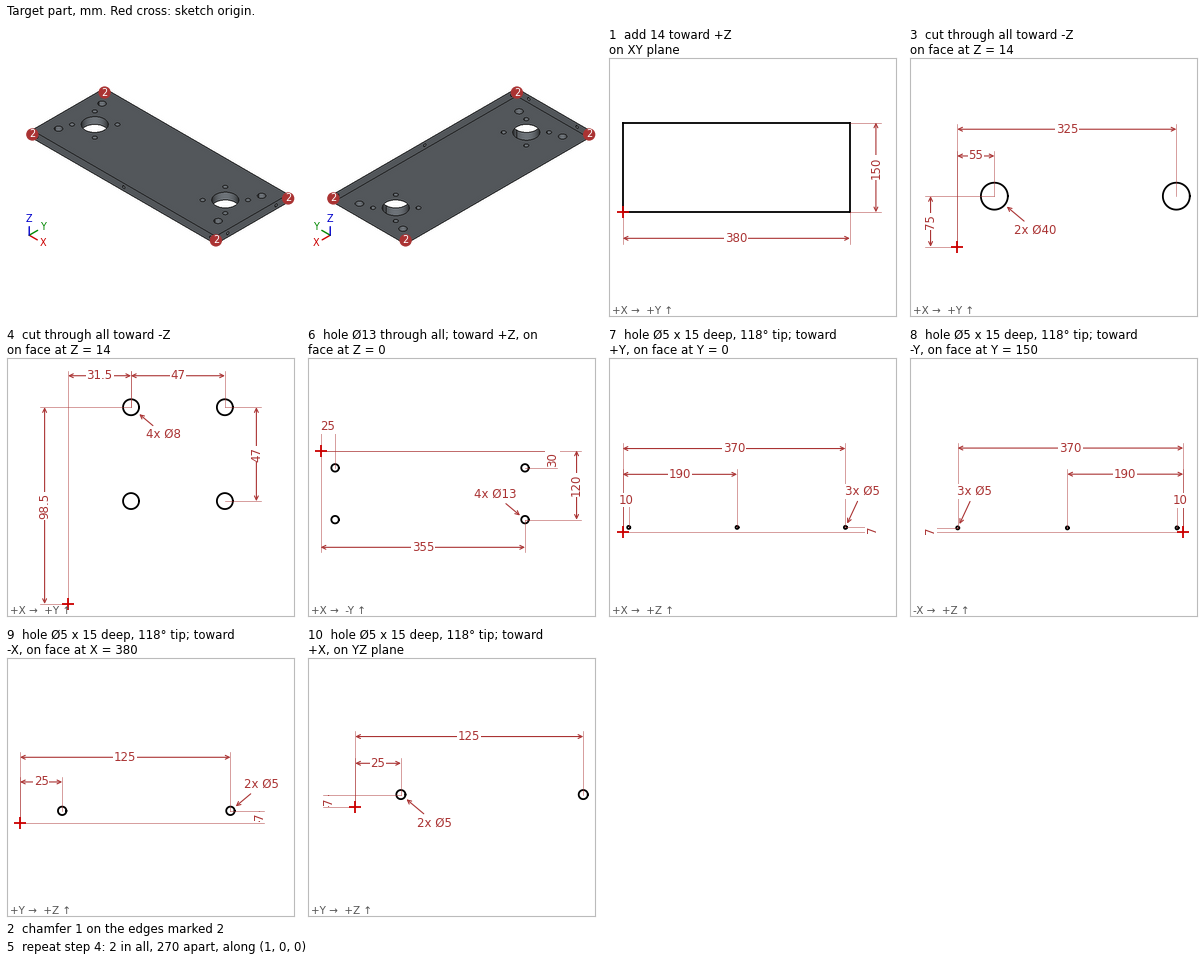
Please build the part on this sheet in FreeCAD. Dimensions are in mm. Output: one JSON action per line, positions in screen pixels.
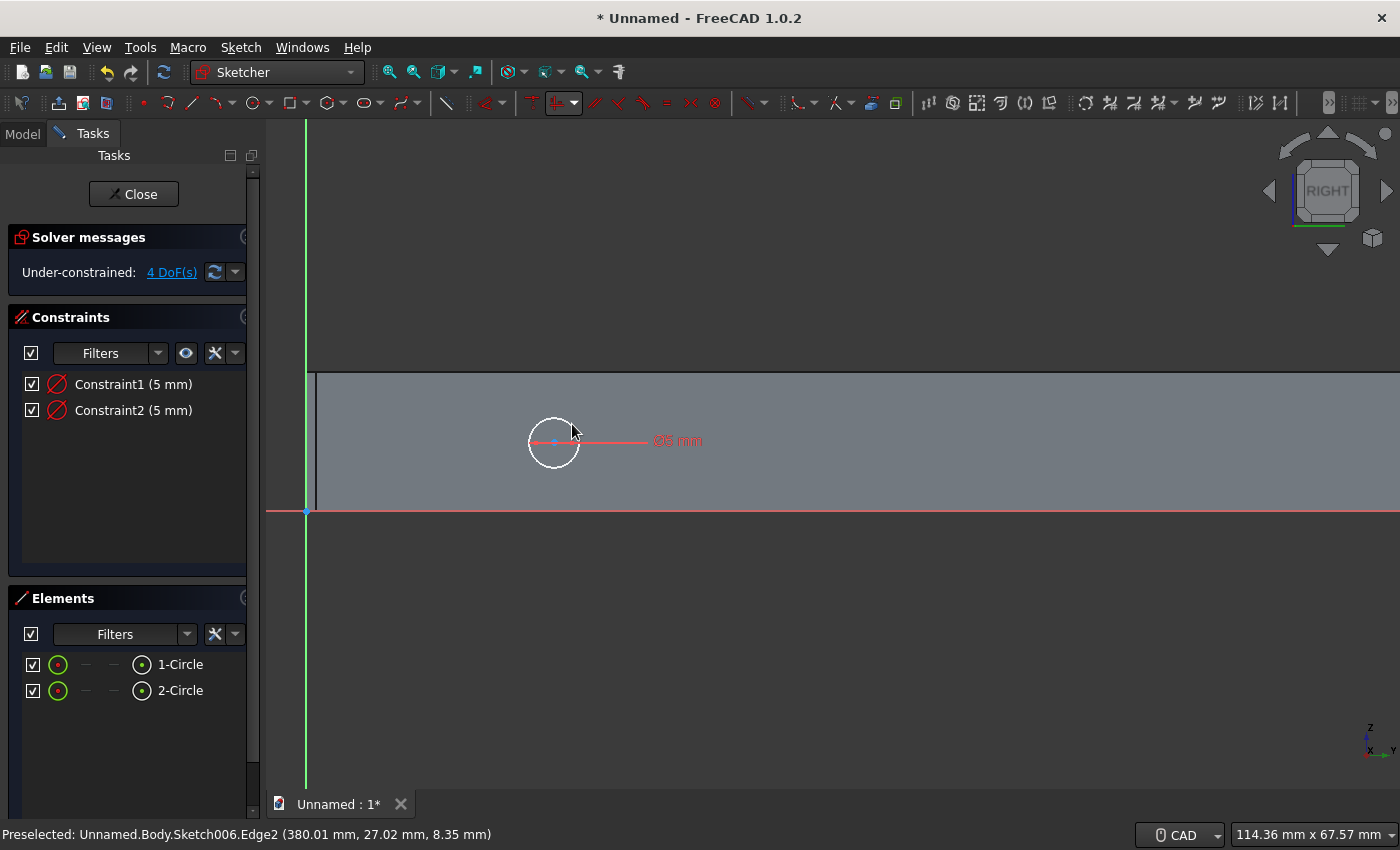
{"action": "scroll", "coordinate": [553, 442], "scroll_direction": "down", "scroll_amount": 3}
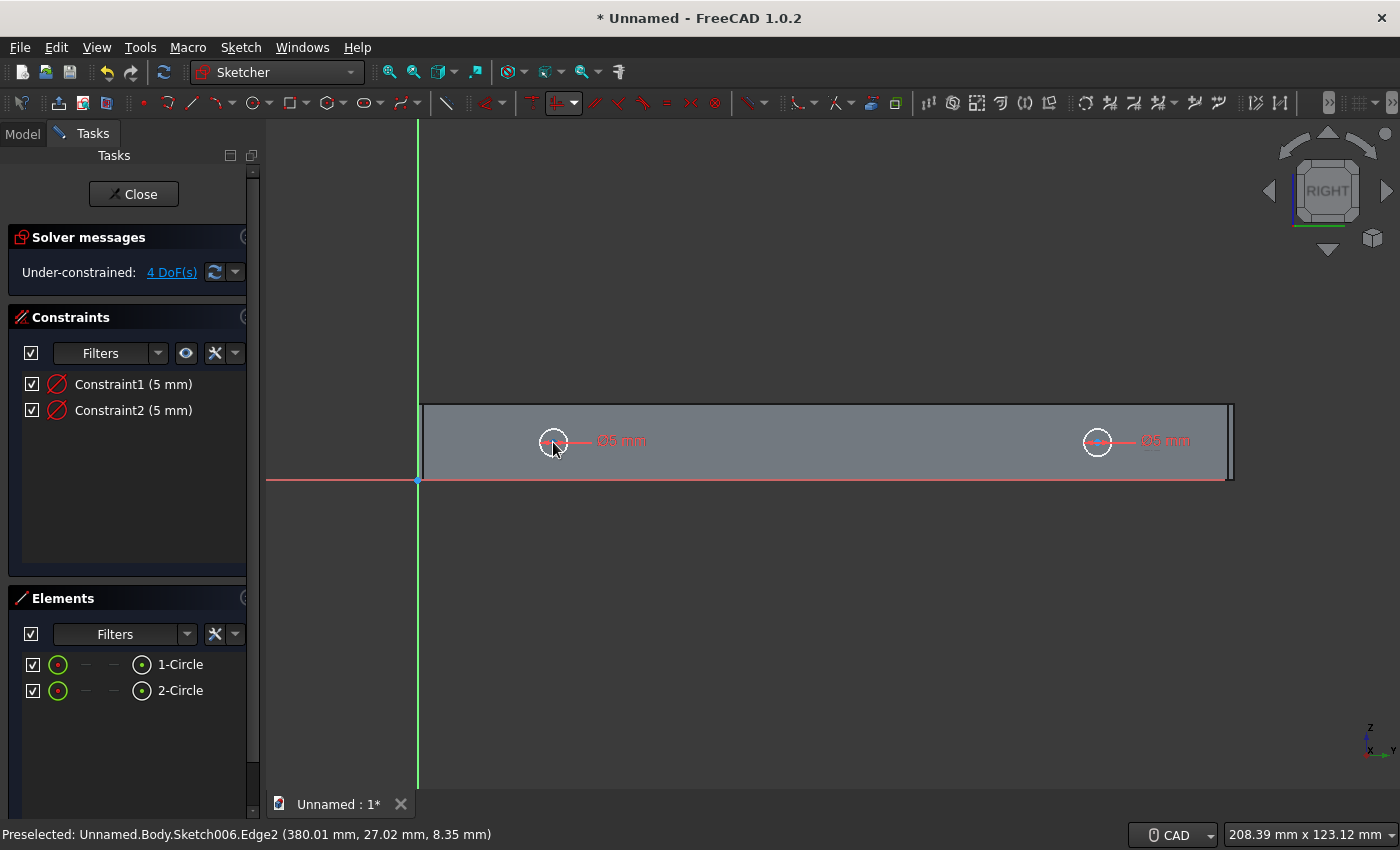
{"action": "left_click", "coordinate": [1098, 443]}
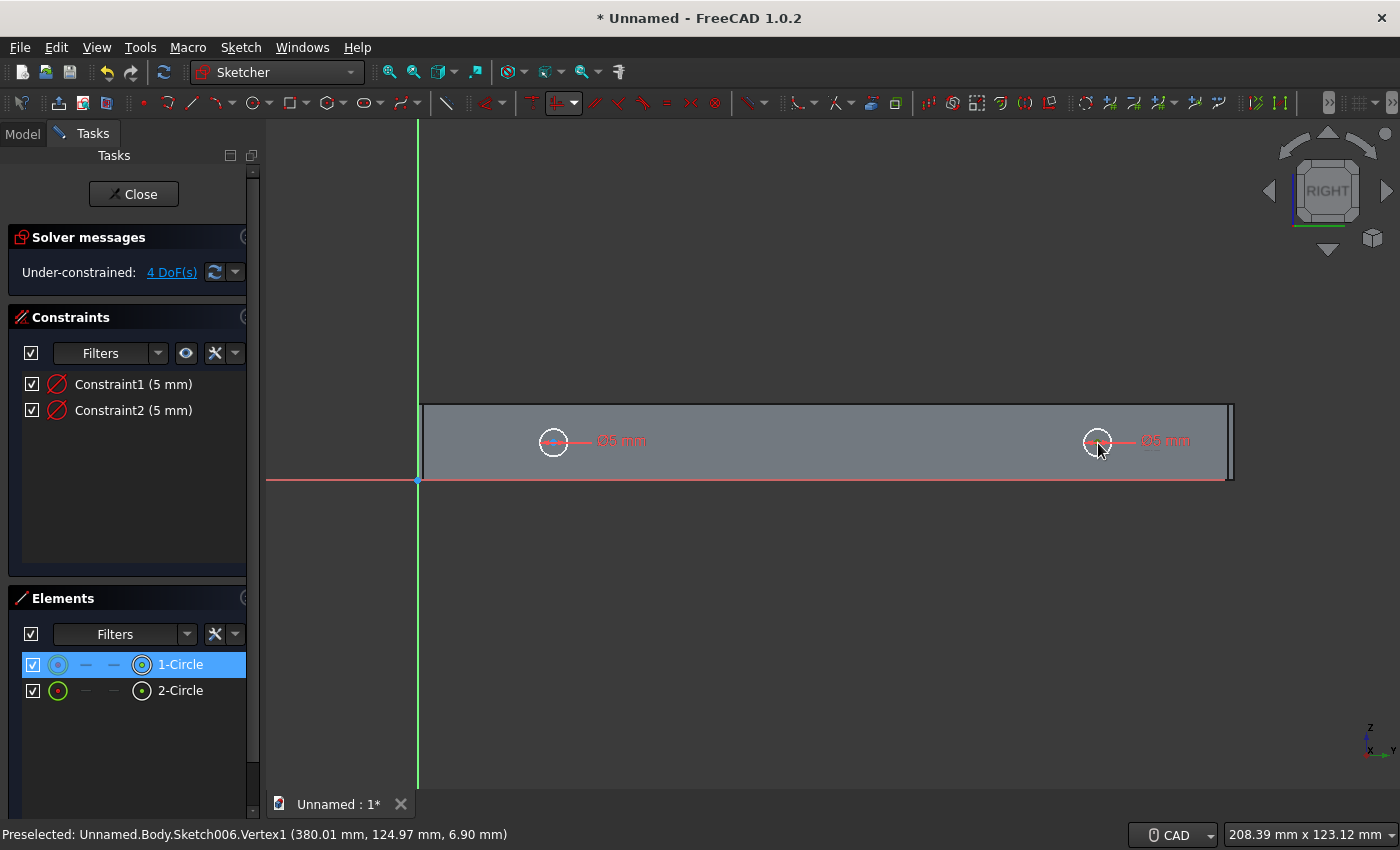
{"action": "left_click", "coordinate": [554, 443]}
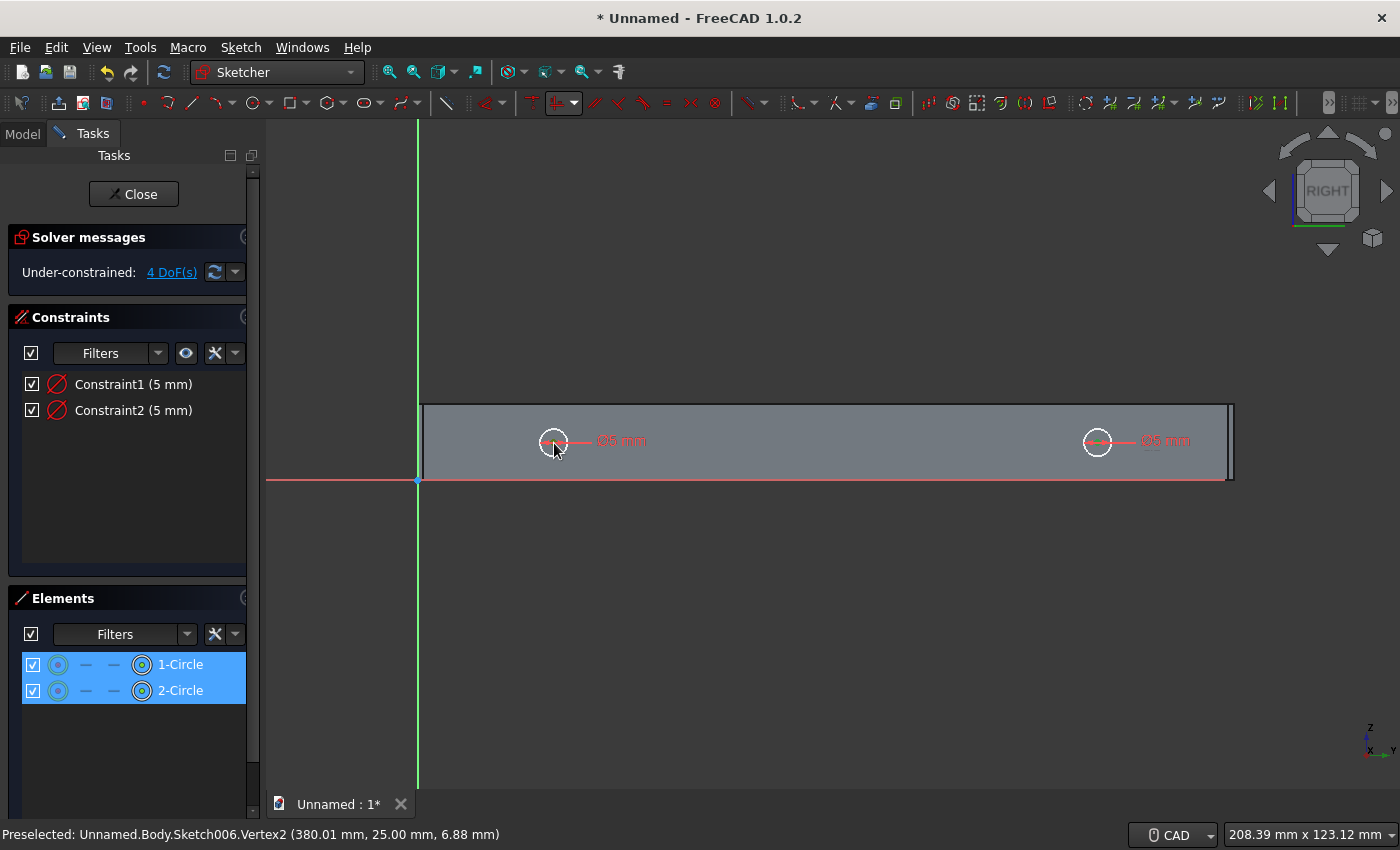
{"action": "key", "text": "h"}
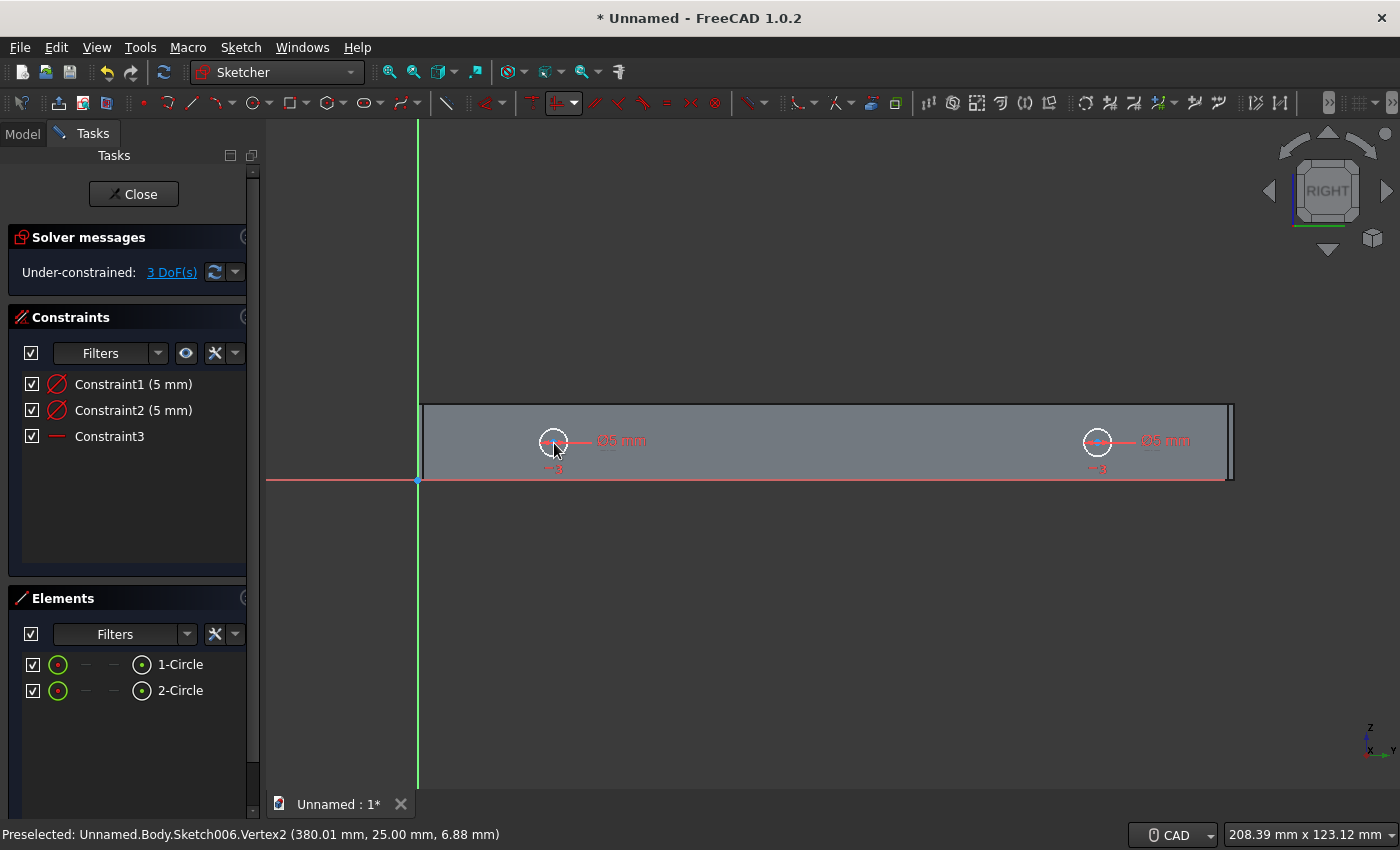
{"action": "key", "text": "d"}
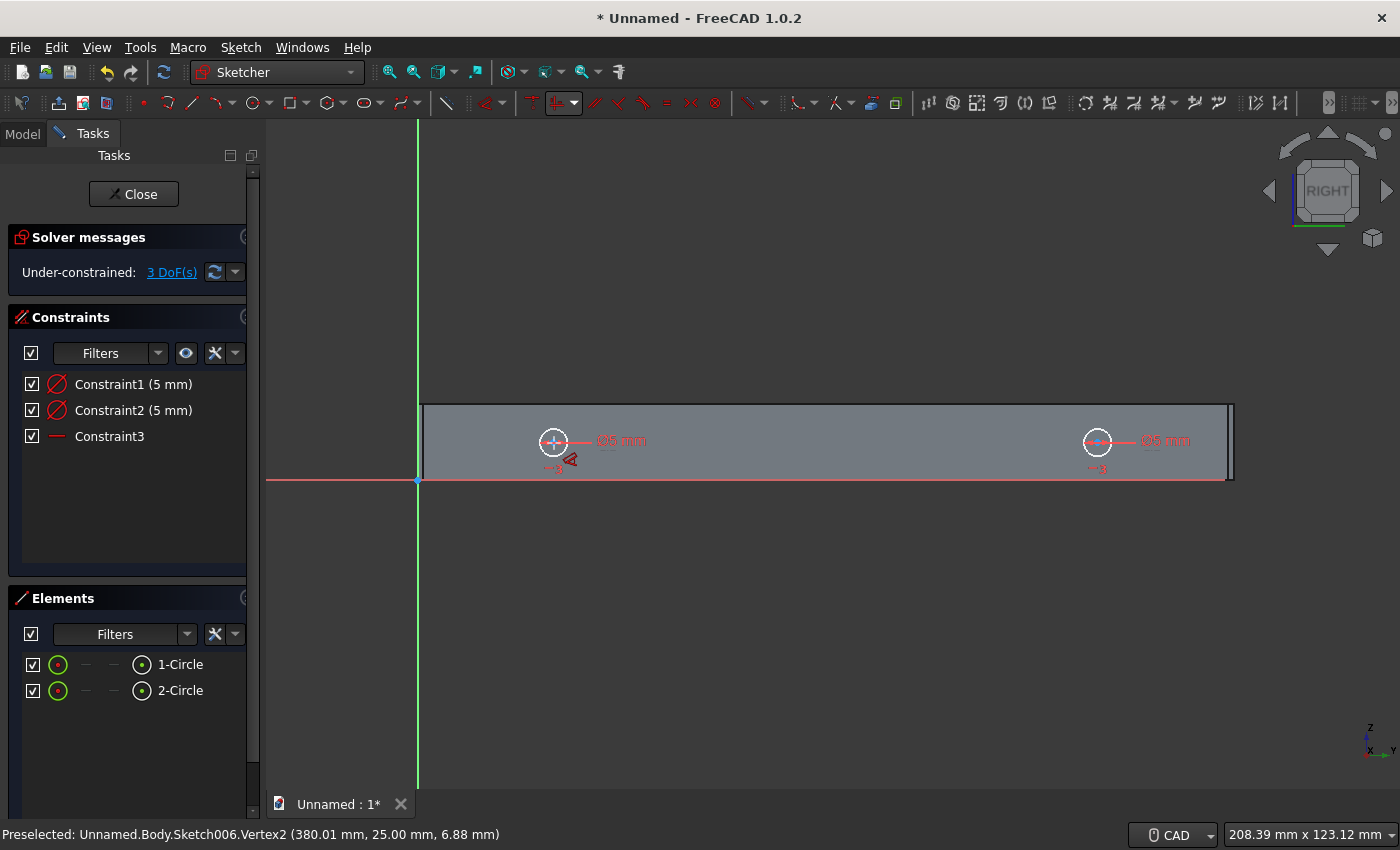
{"action": "left_click", "coordinate": [1098, 443]}
{"action": "left_click", "coordinate": [384, 461]}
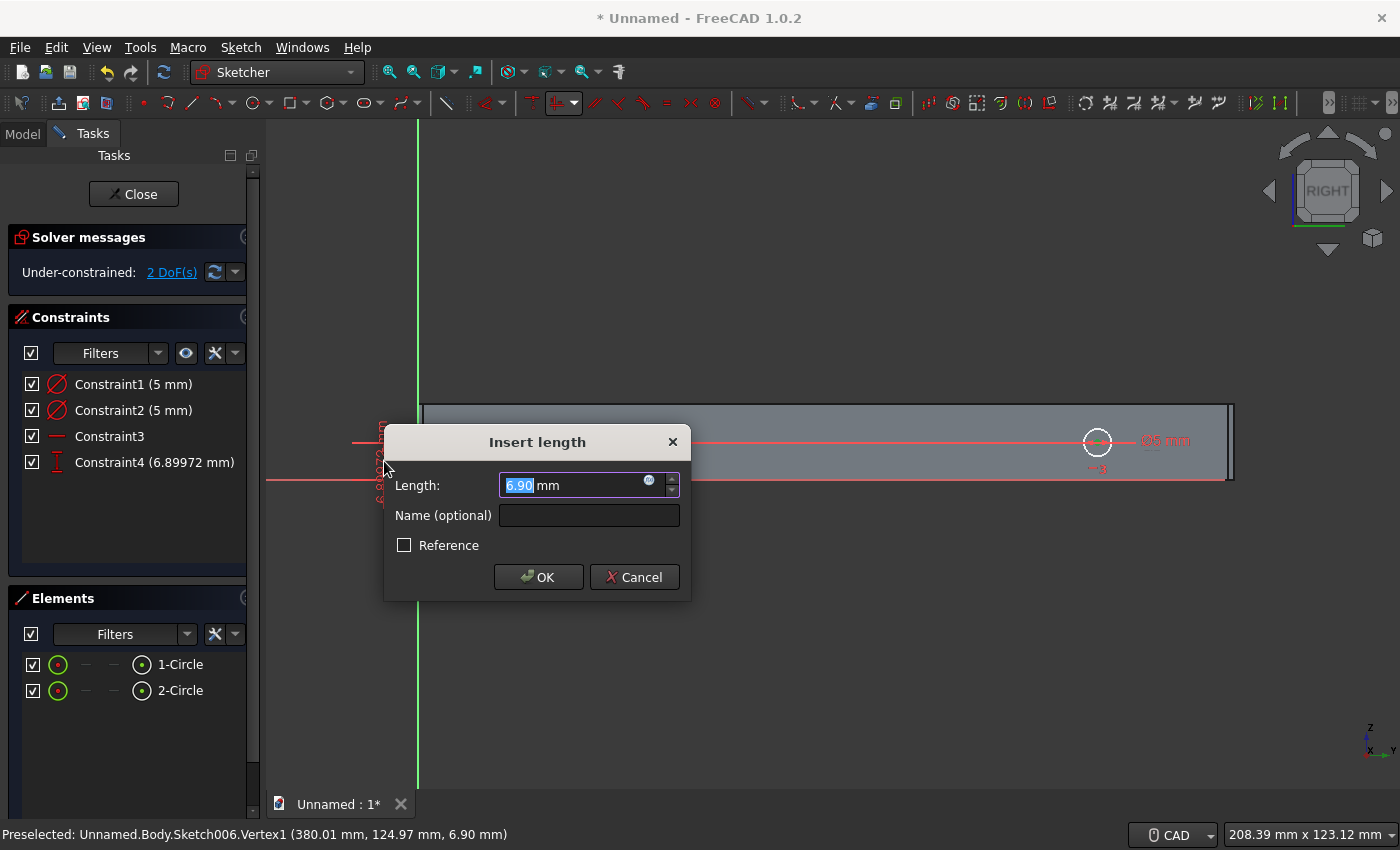
{"action": "type", "text": "7"}
{"action": "key", "text": "Return"}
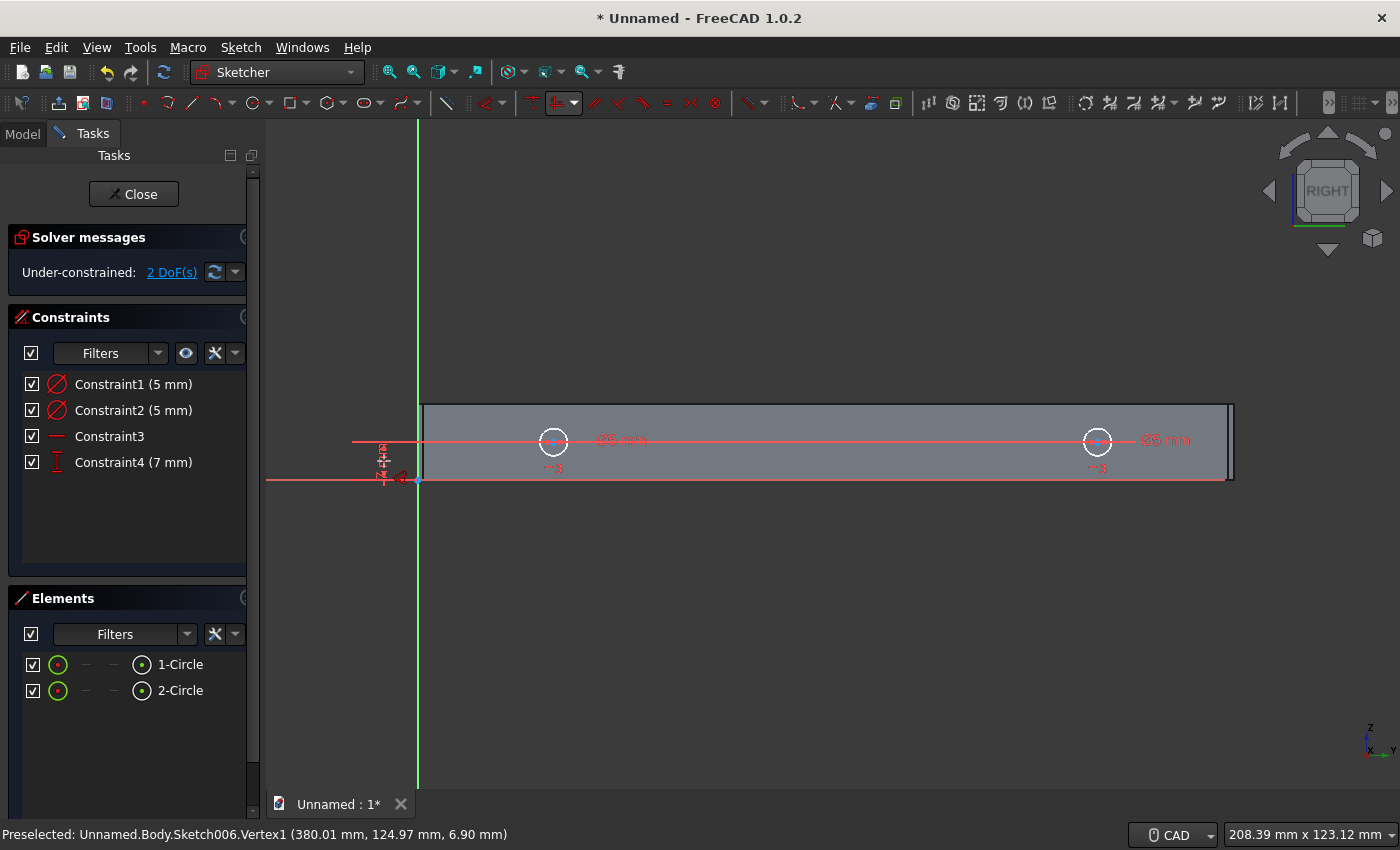
{"action": "left_click", "coordinate": [554, 442]}
{"action": "left_click", "coordinate": [486, 514]}